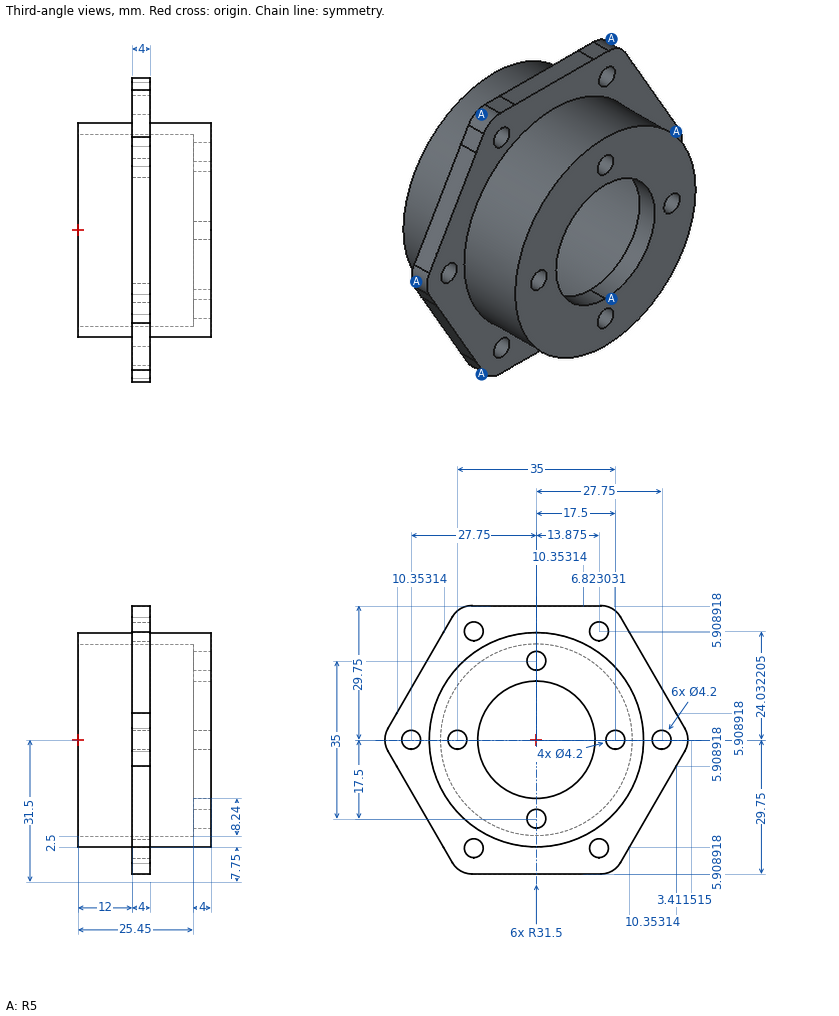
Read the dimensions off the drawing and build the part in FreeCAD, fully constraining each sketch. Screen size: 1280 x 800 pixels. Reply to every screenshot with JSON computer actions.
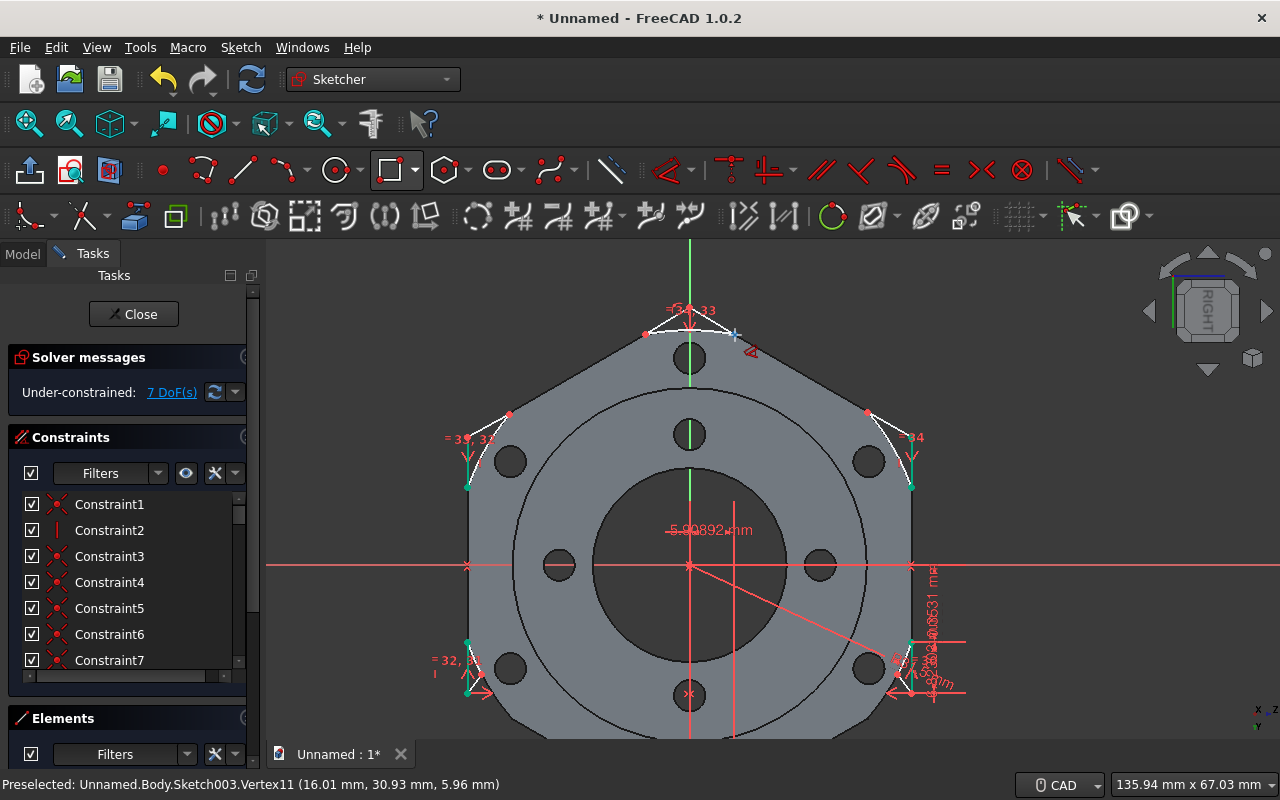
{"action": "left_click", "coordinate": [734, 335]}
{"action": "left_click", "coordinate": [712, 301]}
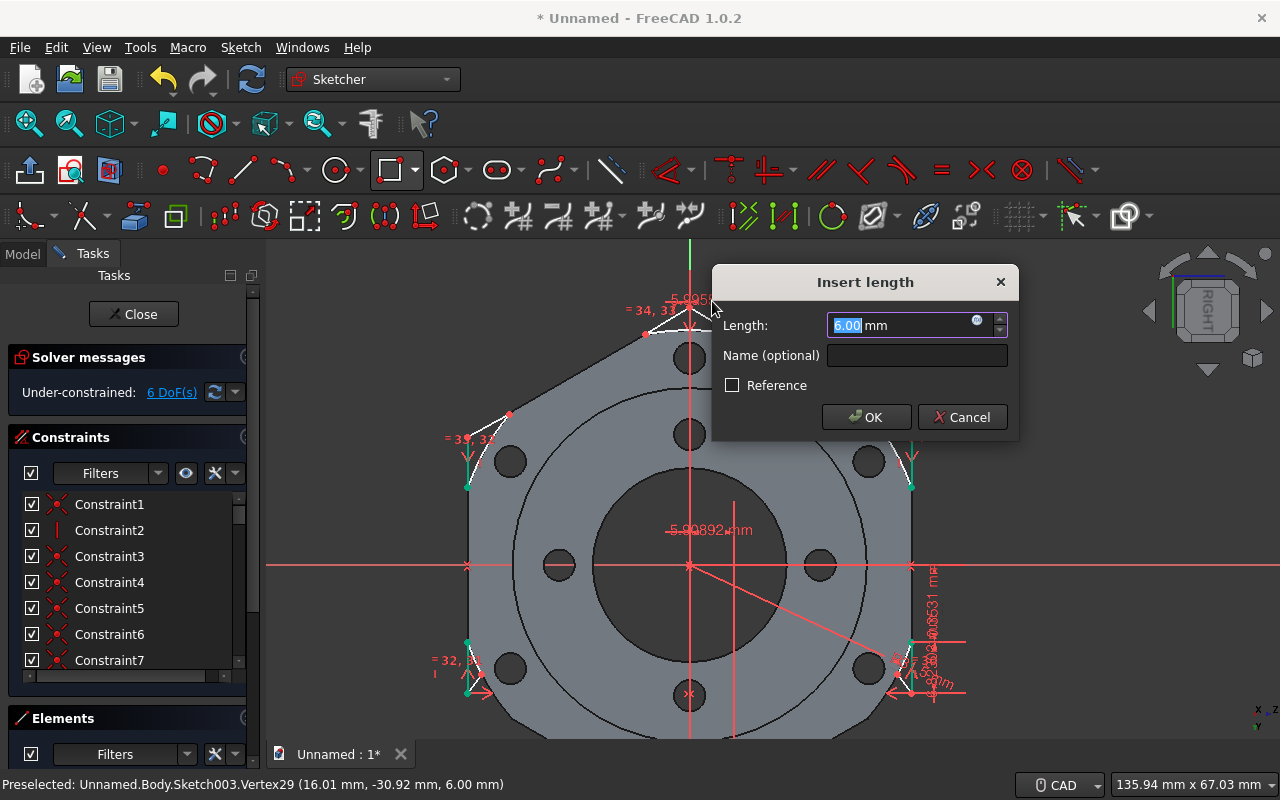
{"action": "type", "text": "5.908918"}
{"action": "key", "text": "Return"}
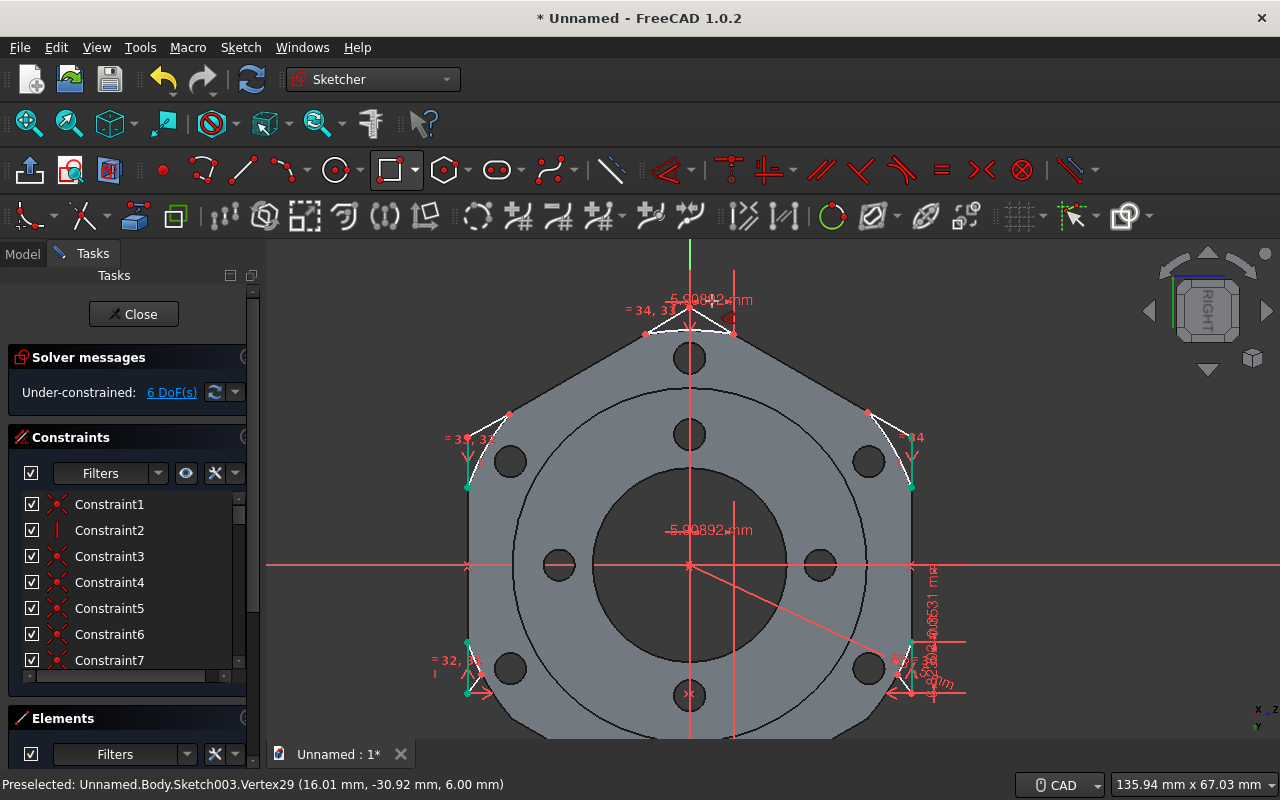
{"action": "left_click", "coordinate": [645, 334]}
{"action": "left_click", "coordinate": [667, 599]}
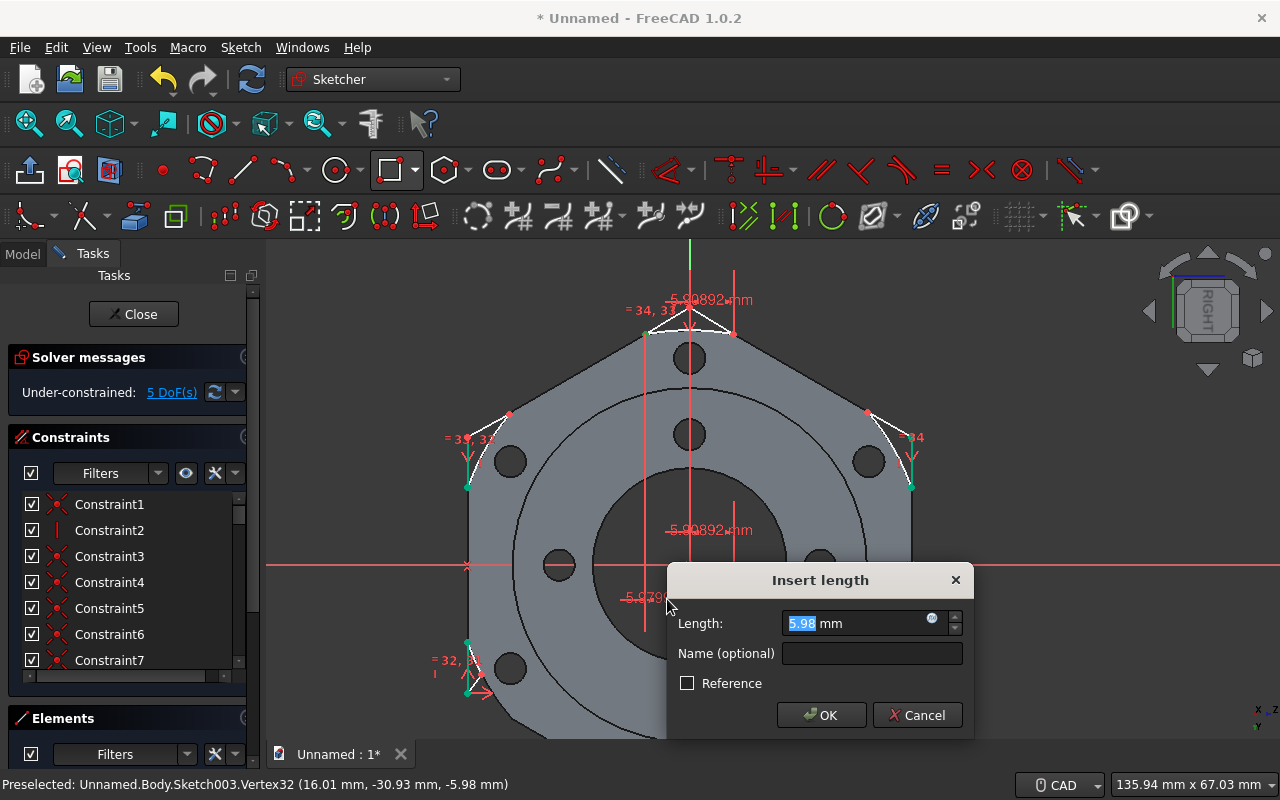
{"action": "type", "text": "5.908918"}
{"action": "key", "text": "Return"}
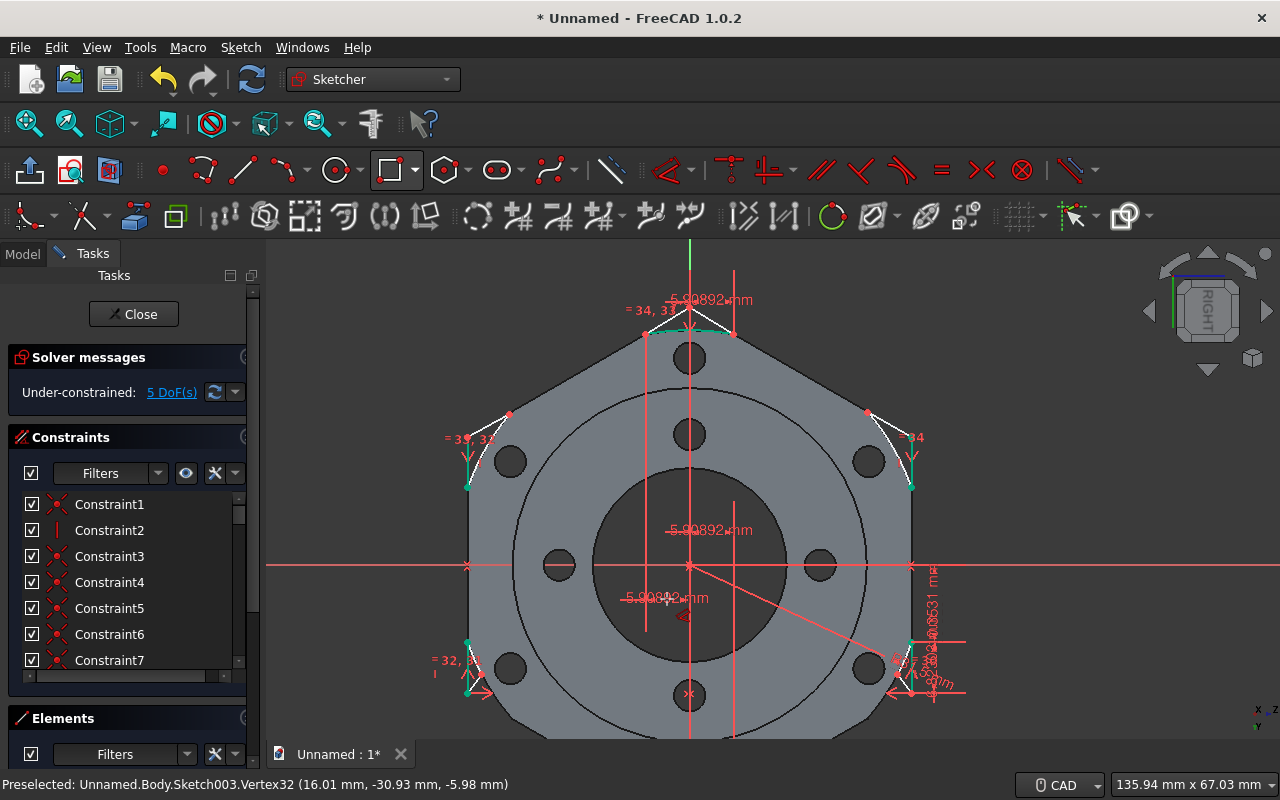
{"action": "scroll", "coordinate": [903, 682], "scroll_direction": "up", "scroll_amount": 3}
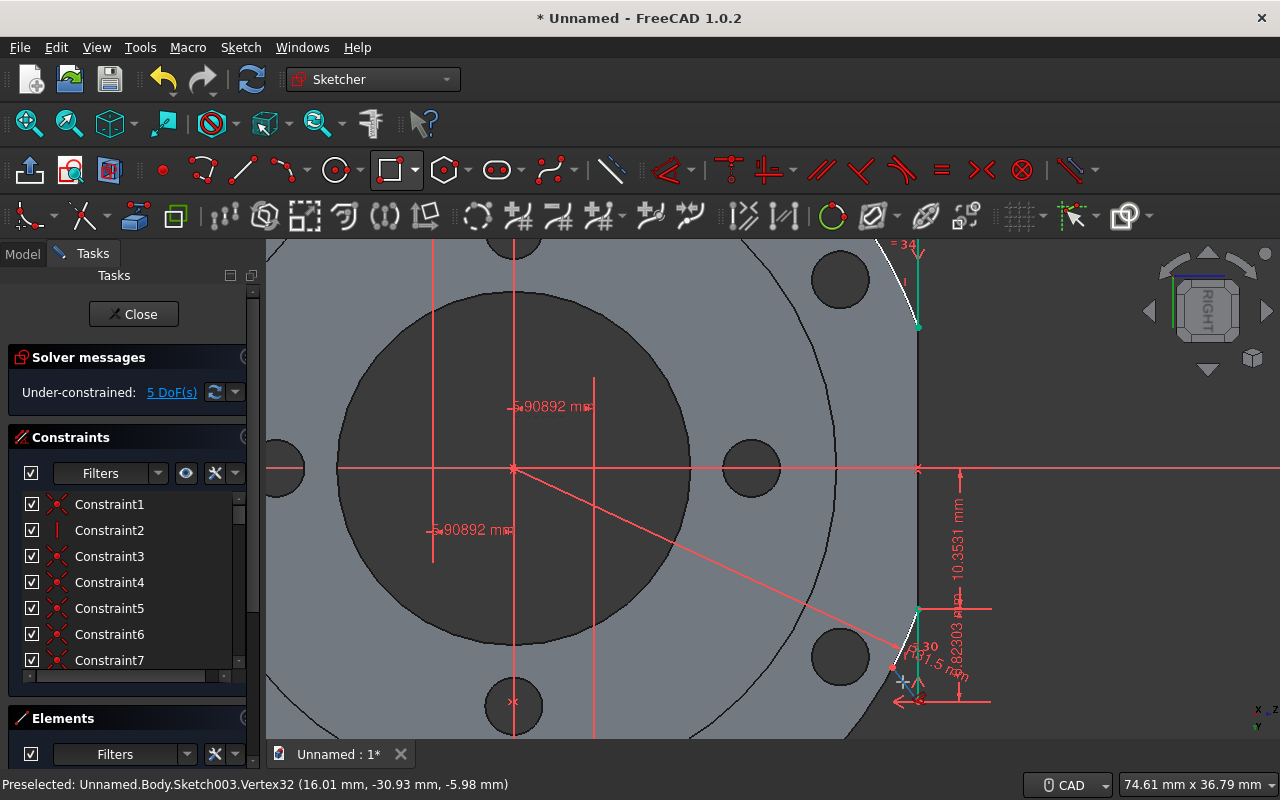
{"action": "left_click", "coordinate": [903, 681]}
{"action": "left_click", "coordinate": [900, 610]}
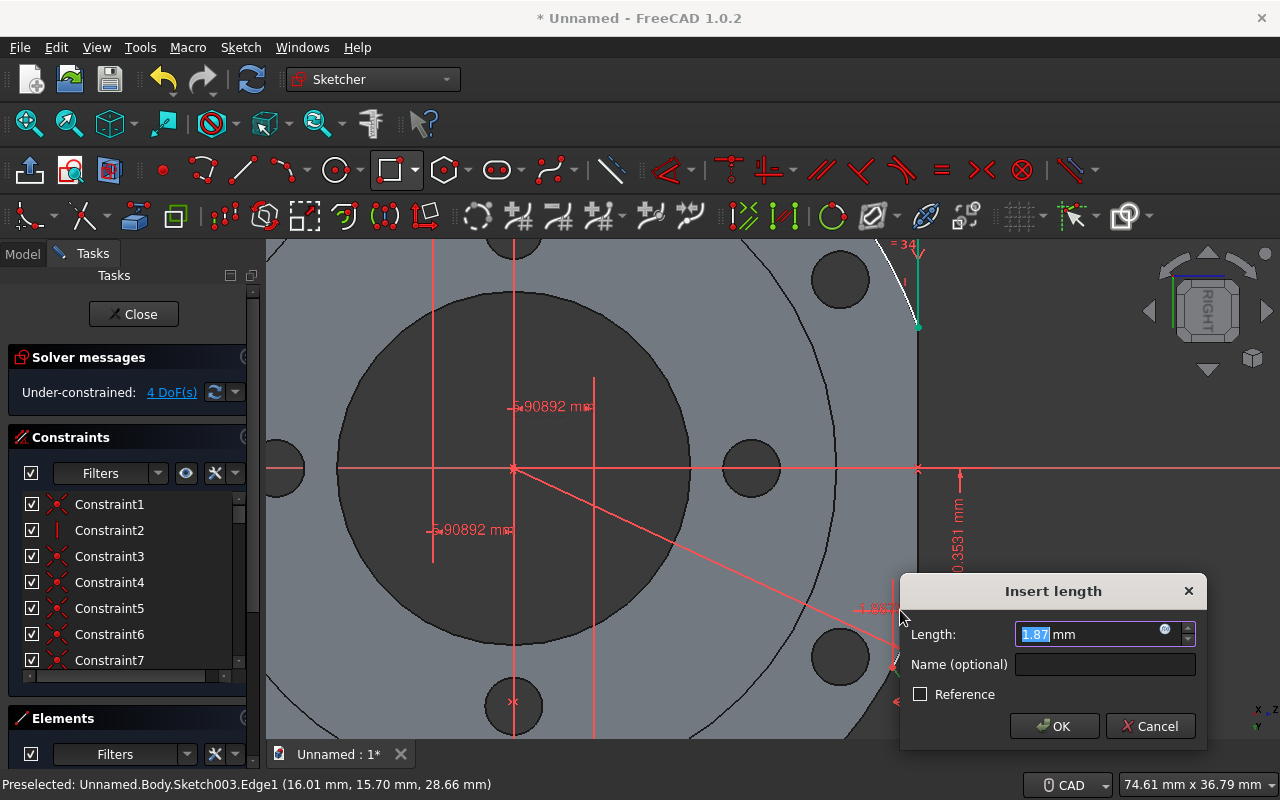
{"action": "type", "text": "5.908918"}
{"action": "key", "text": "Return"}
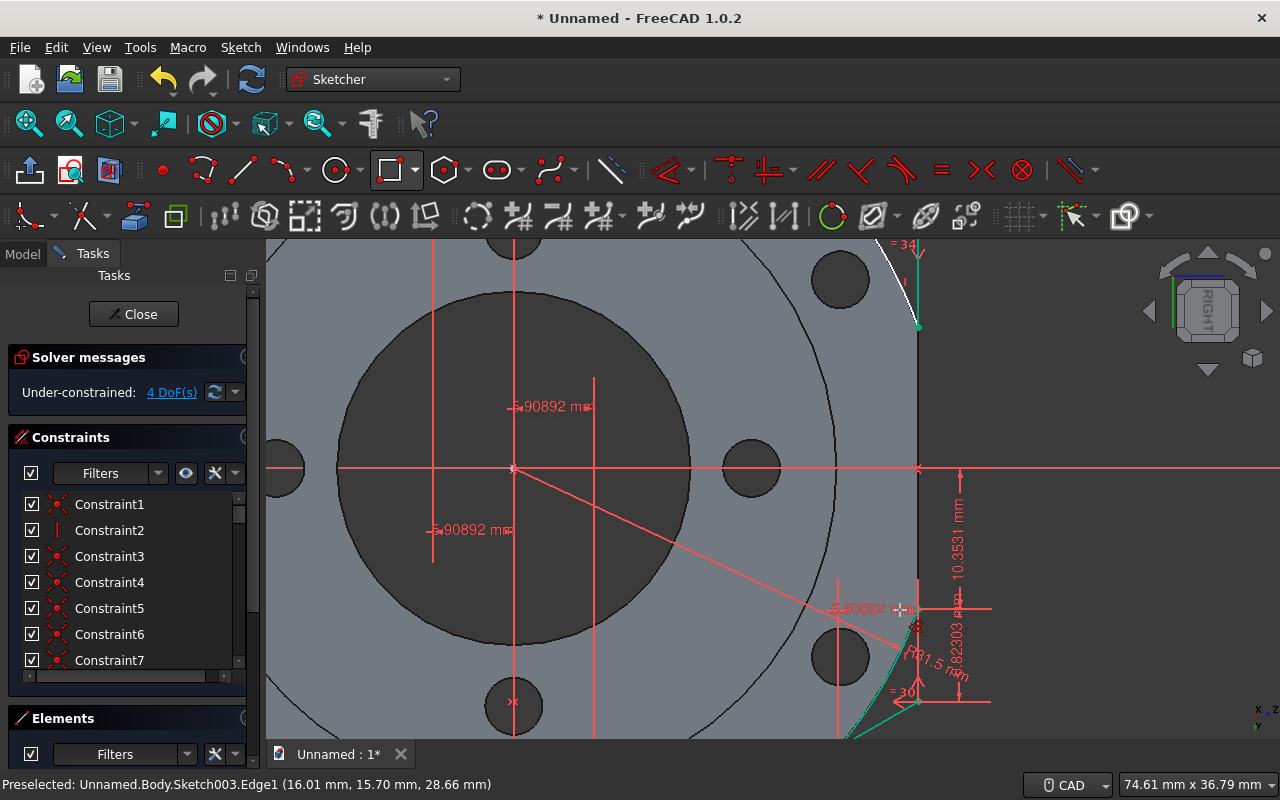
{"action": "scroll", "coordinate": [815, 501], "scroll_direction": "down", "scroll_amount": 5}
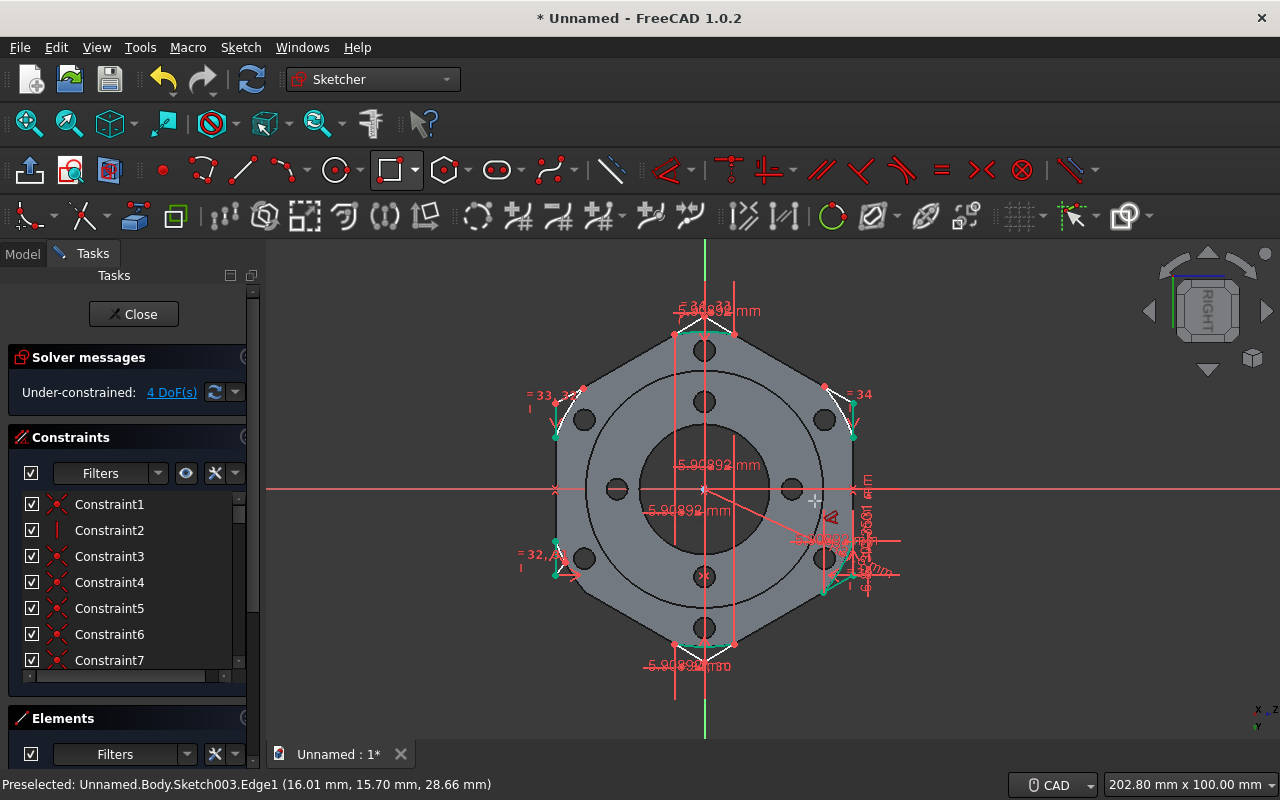
{"action": "scroll", "coordinate": [684, 649], "scroll_direction": "up", "scroll_amount": 7}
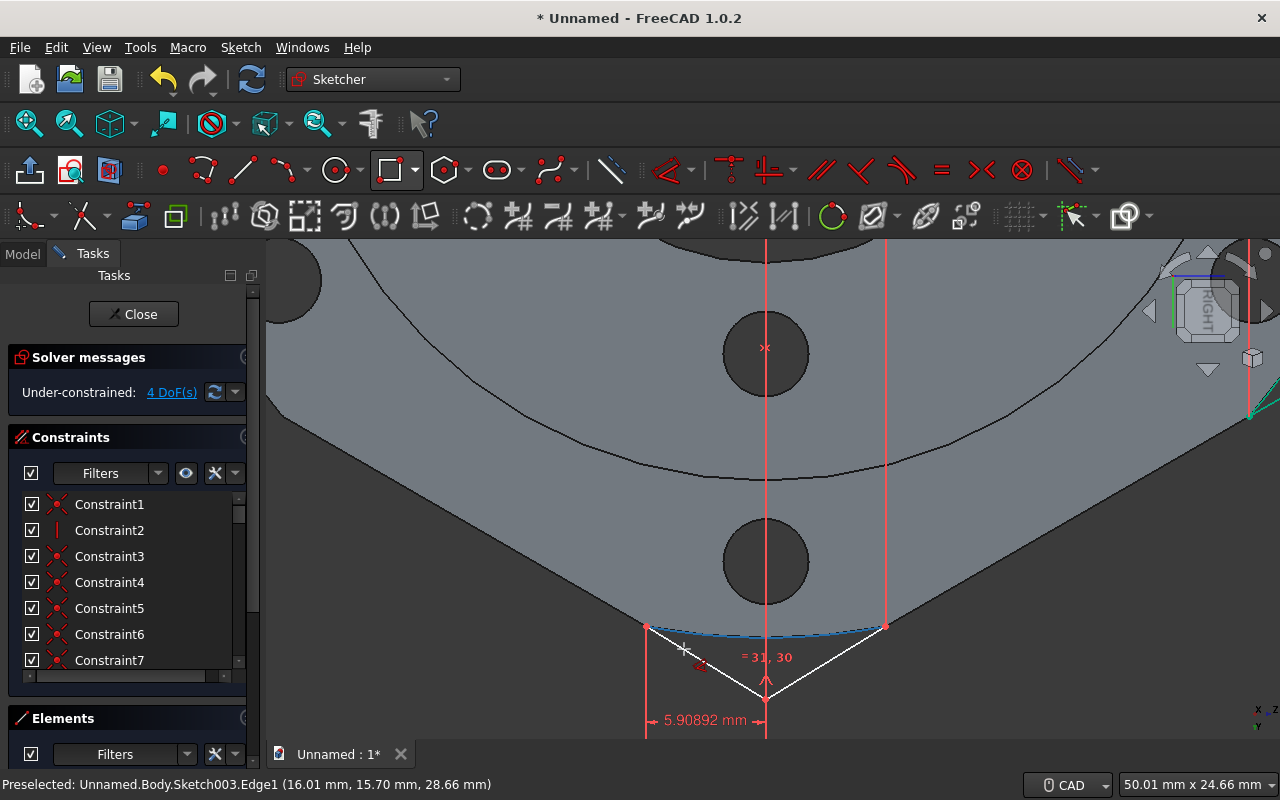
{"action": "left_click", "coordinate": [682, 648]}
{"action": "left_click", "coordinate": [612, 663]}